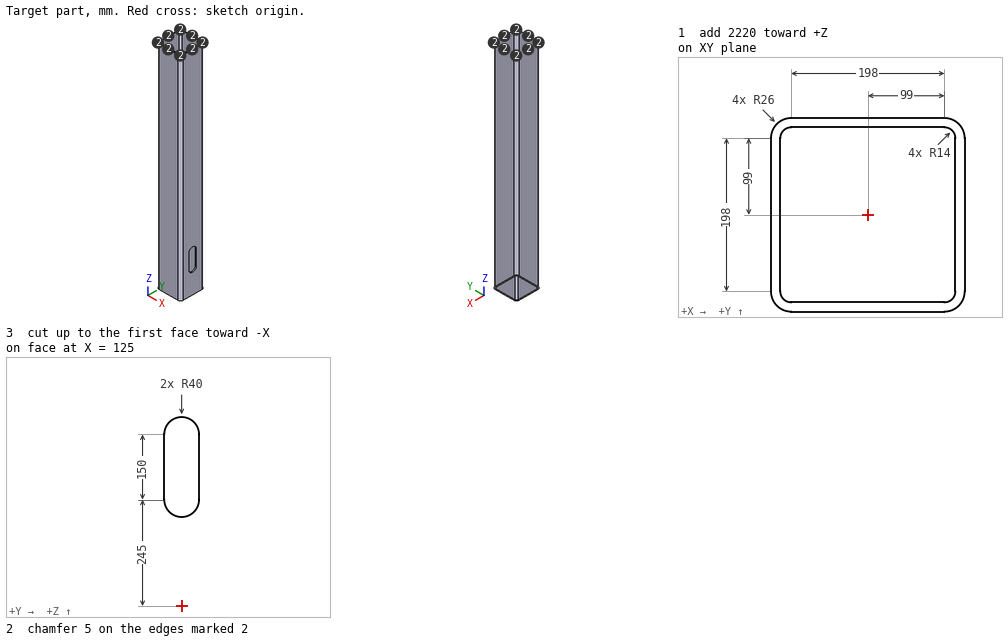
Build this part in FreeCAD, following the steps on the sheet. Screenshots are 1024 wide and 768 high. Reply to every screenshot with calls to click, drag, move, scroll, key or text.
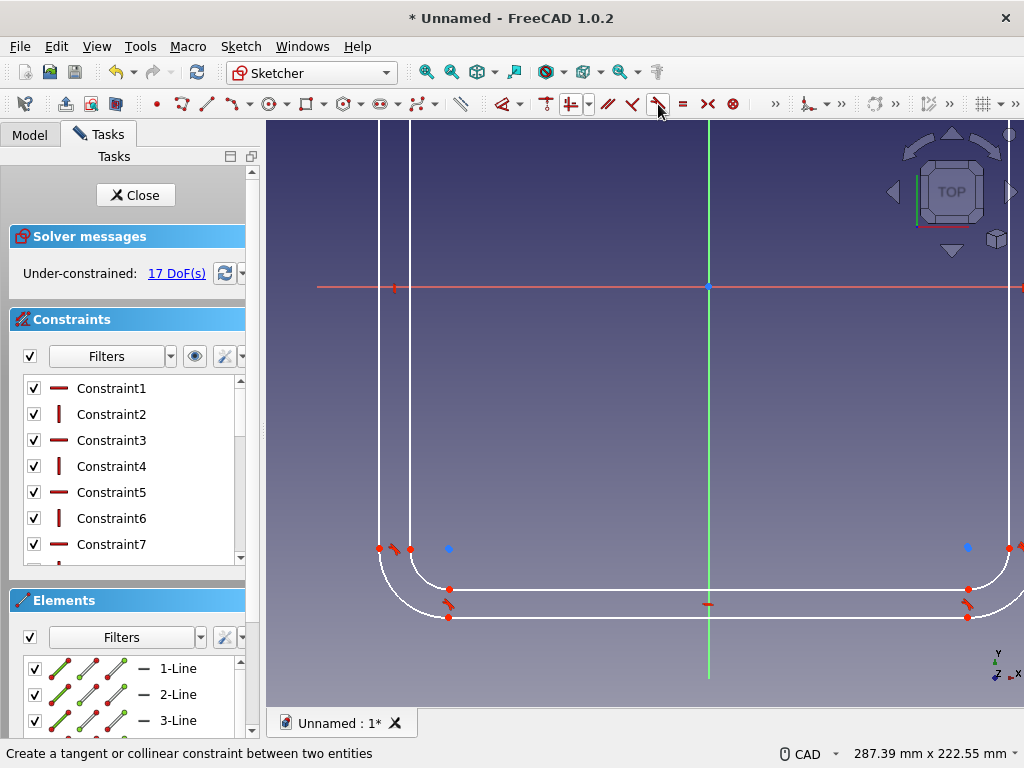
click(410, 393)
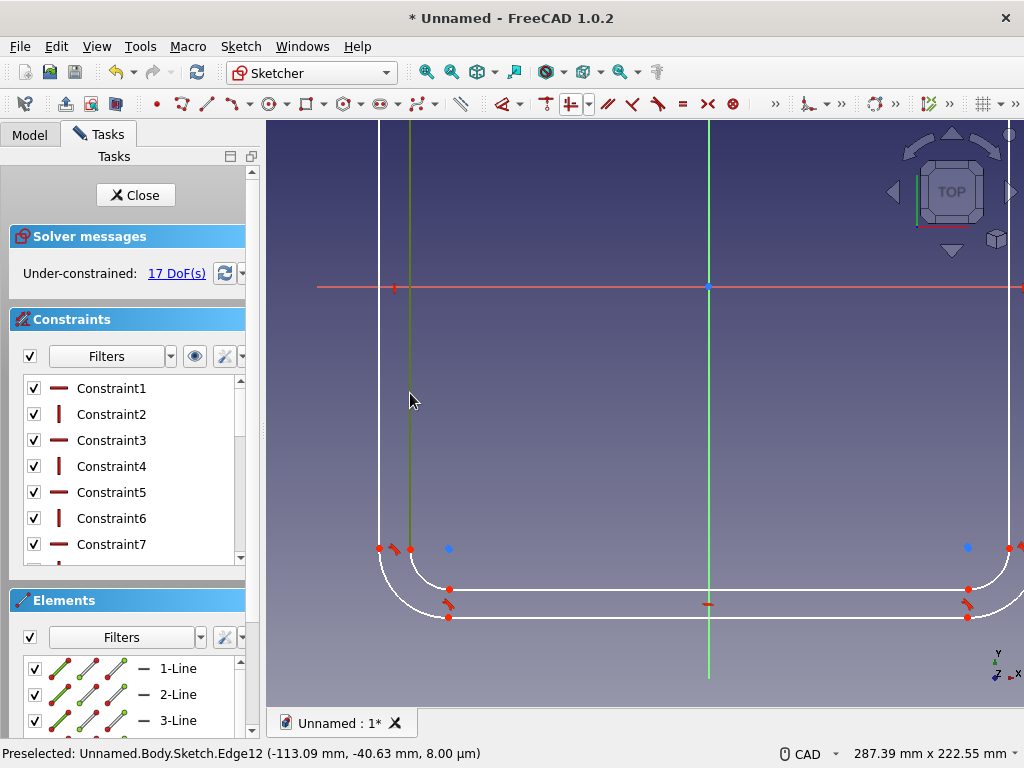
scroll(416, 568, down, 3)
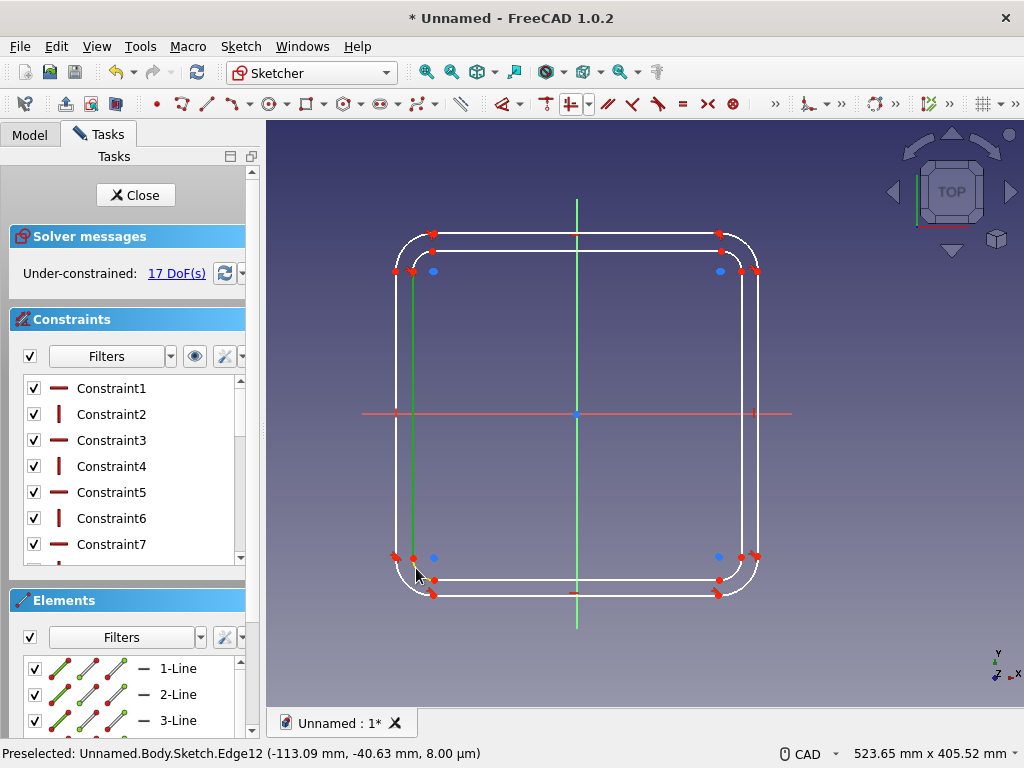
scroll(424, 253, up, 2)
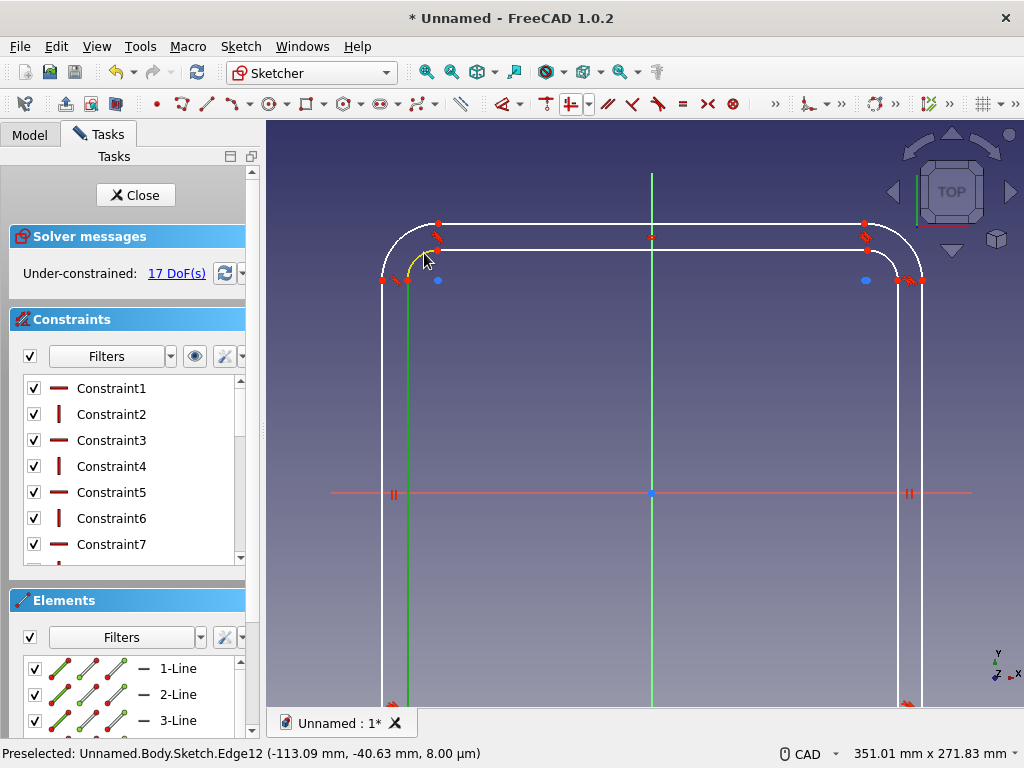
click(424, 254)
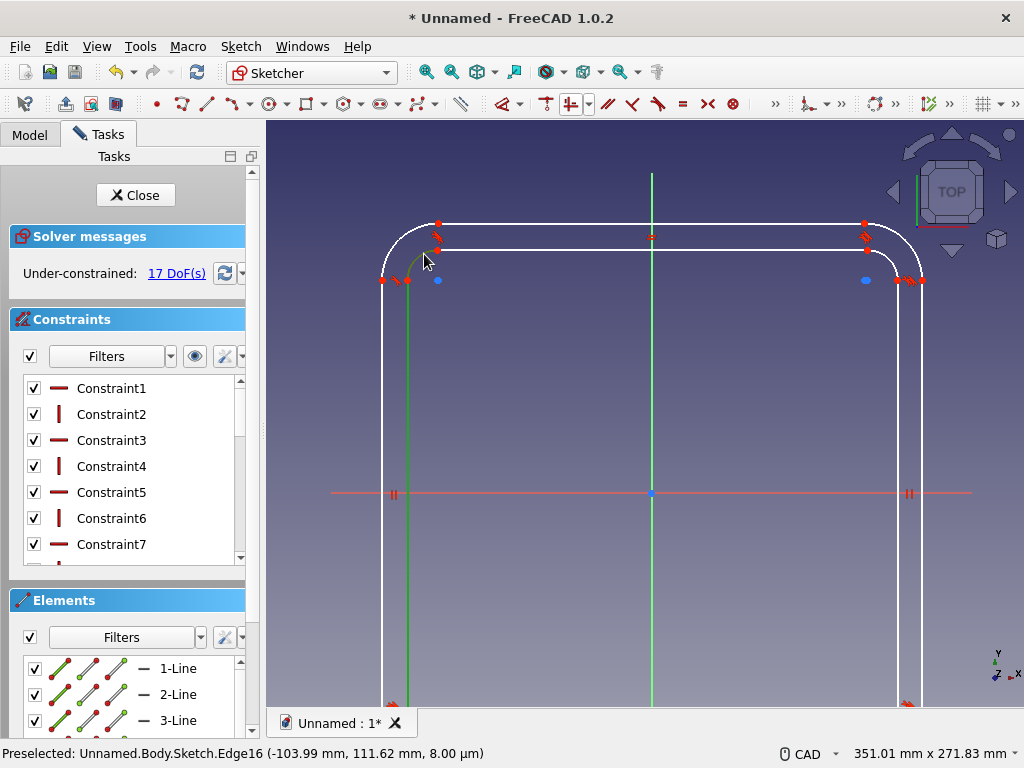
click(658, 104)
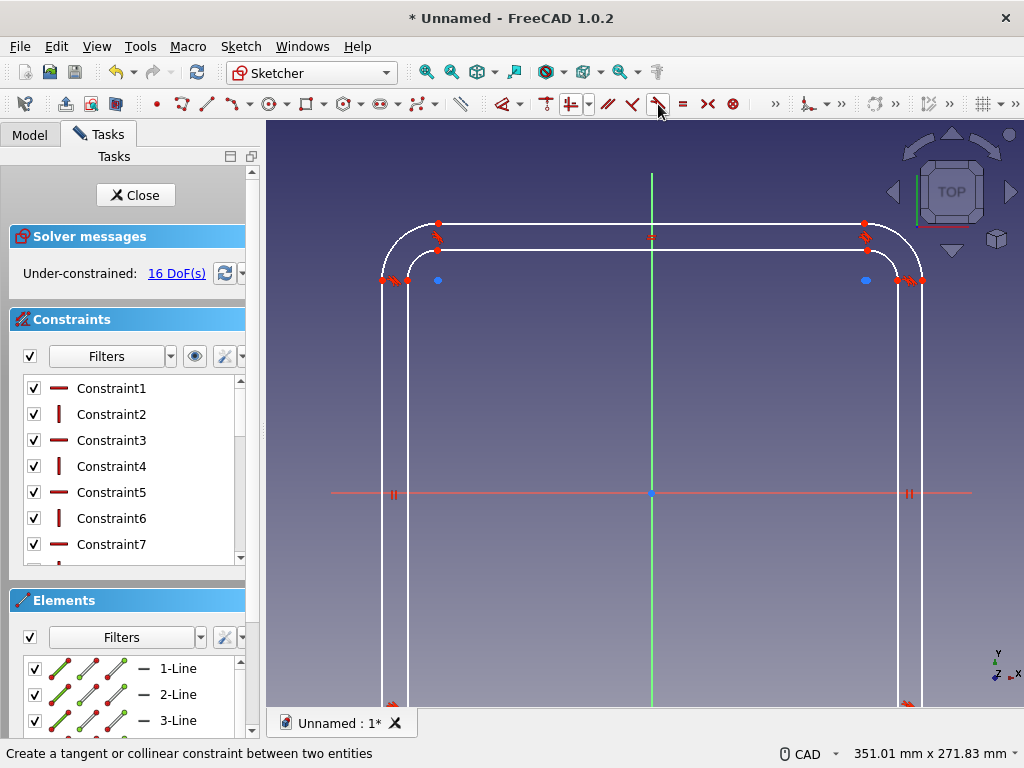
scroll(424, 252, down, 2)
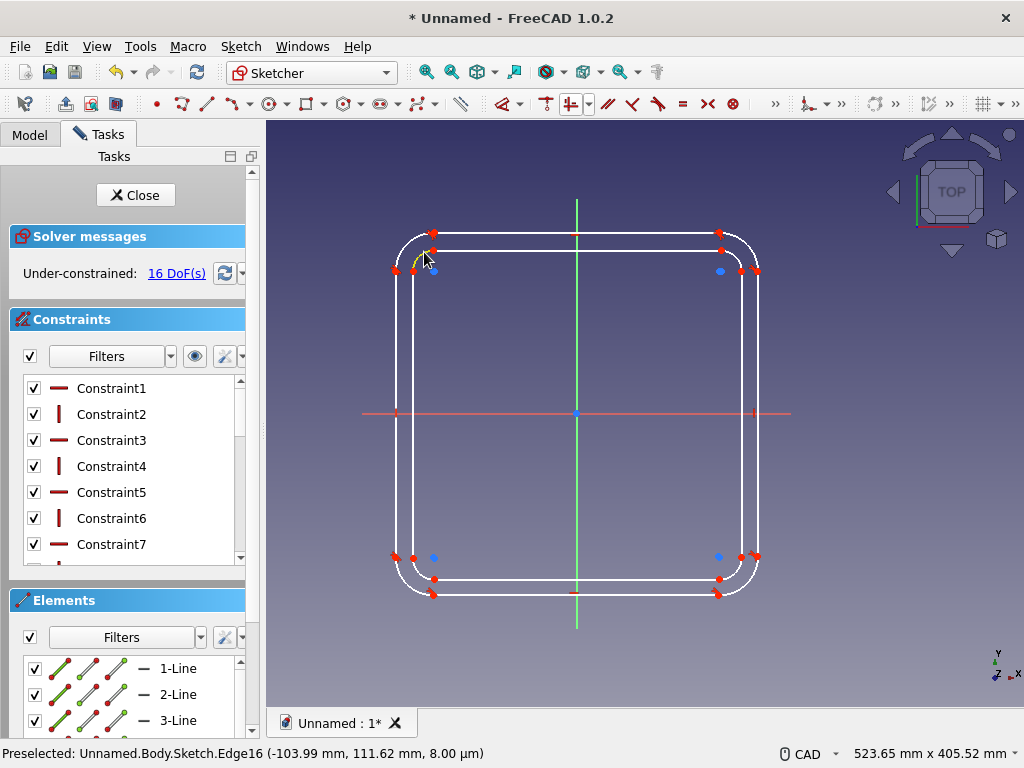
click(754, 254)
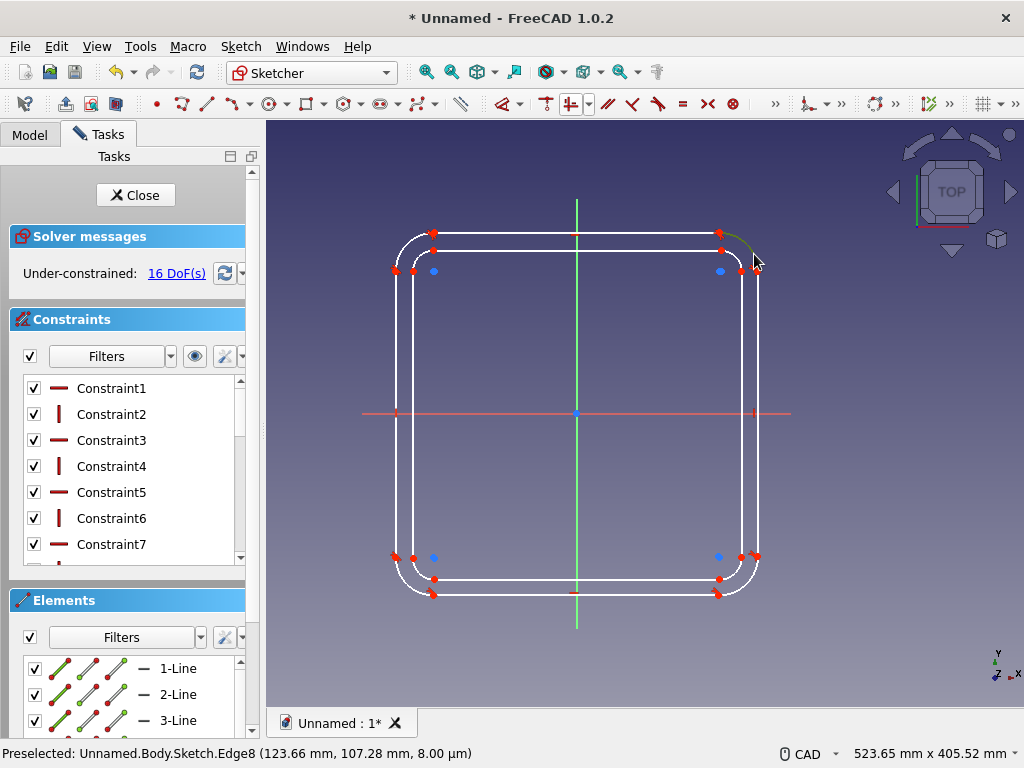
scroll(739, 262, up, 2)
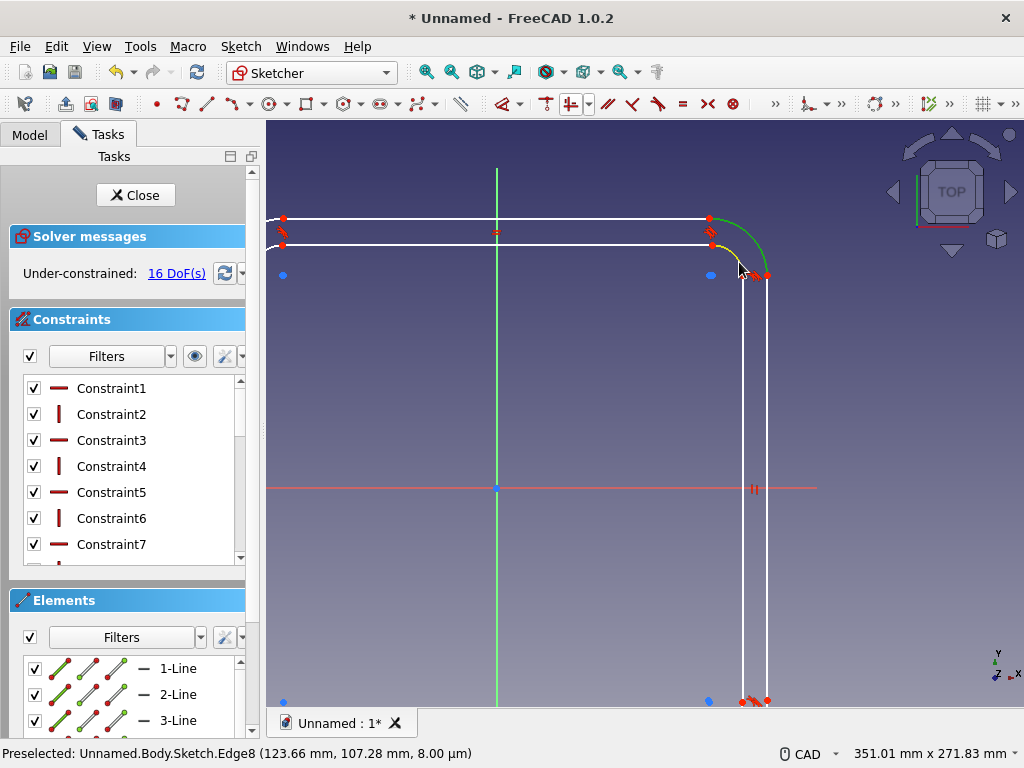
click(739, 262)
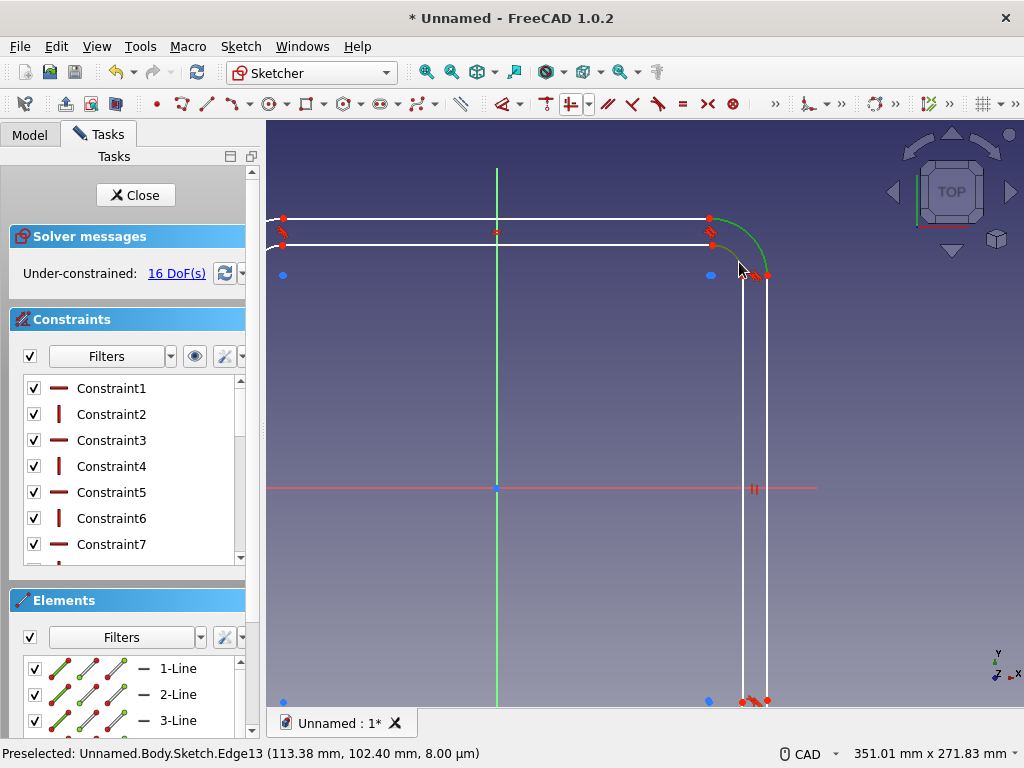
click(546, 104)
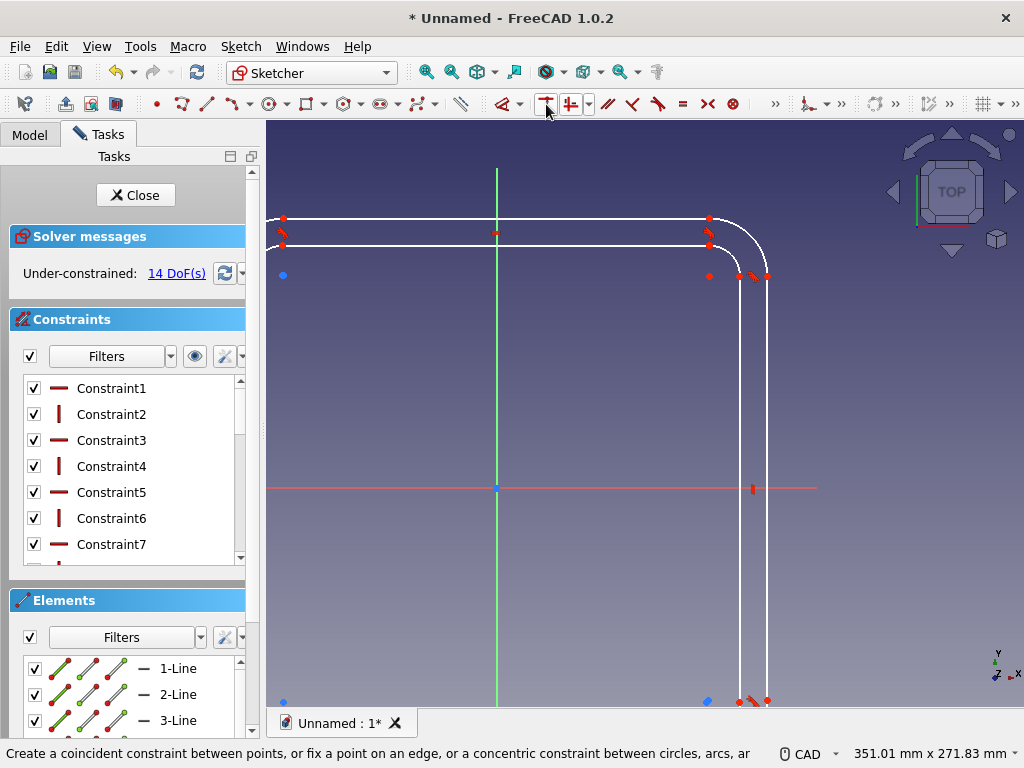
scroll(739, 262, down, 2)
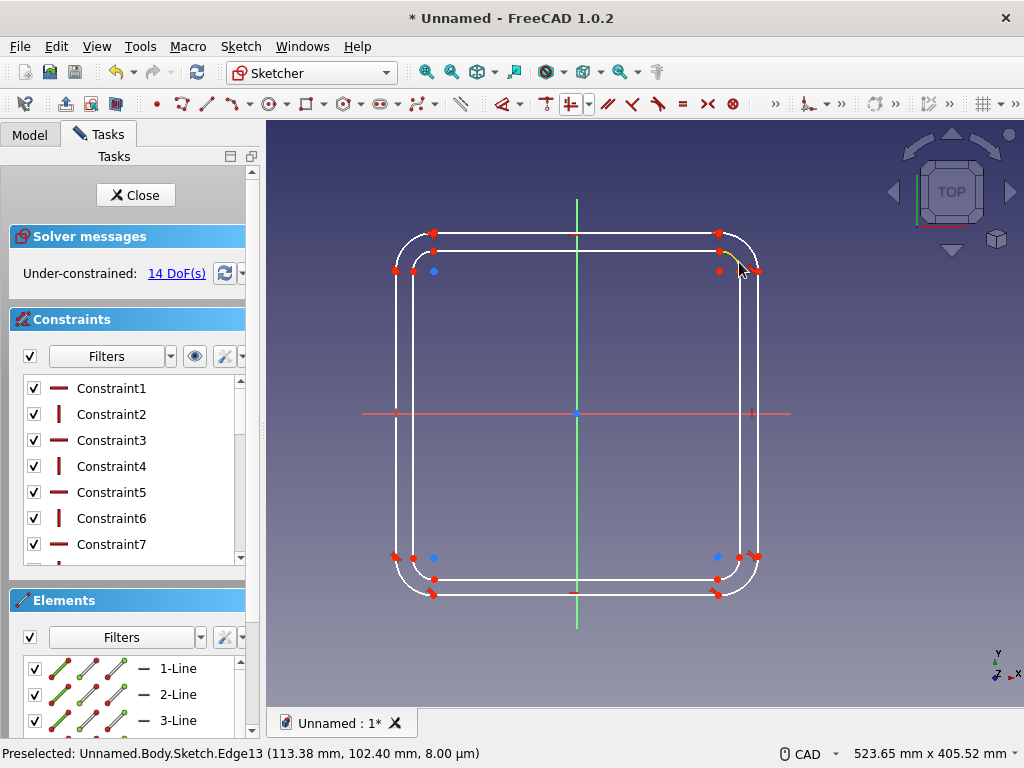
click(737, 591)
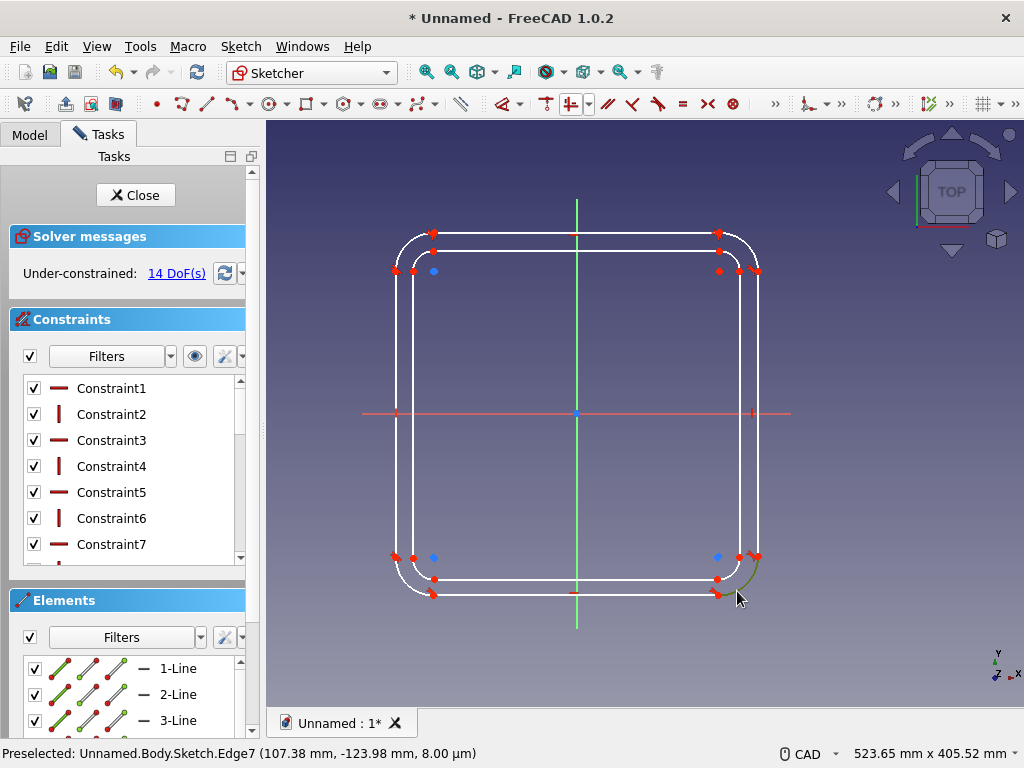
scroll(728, 577, up, 2)